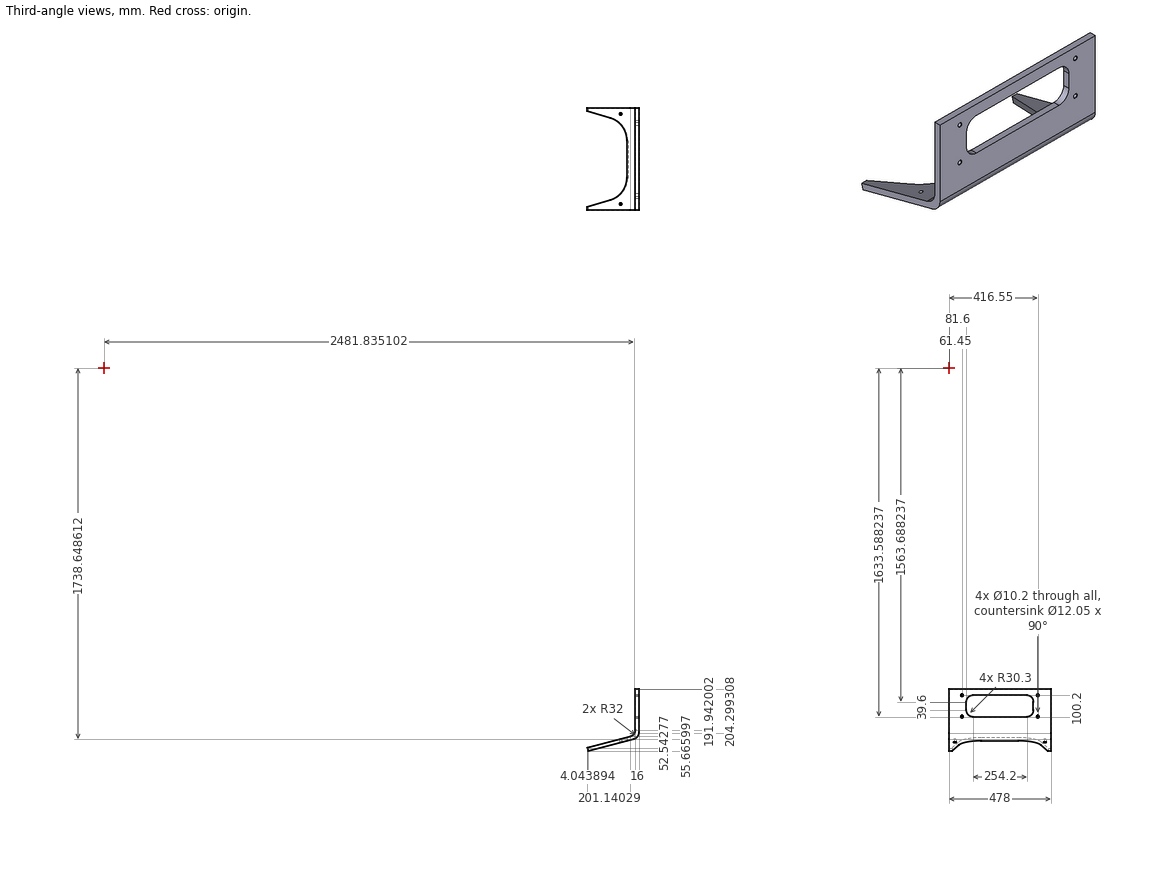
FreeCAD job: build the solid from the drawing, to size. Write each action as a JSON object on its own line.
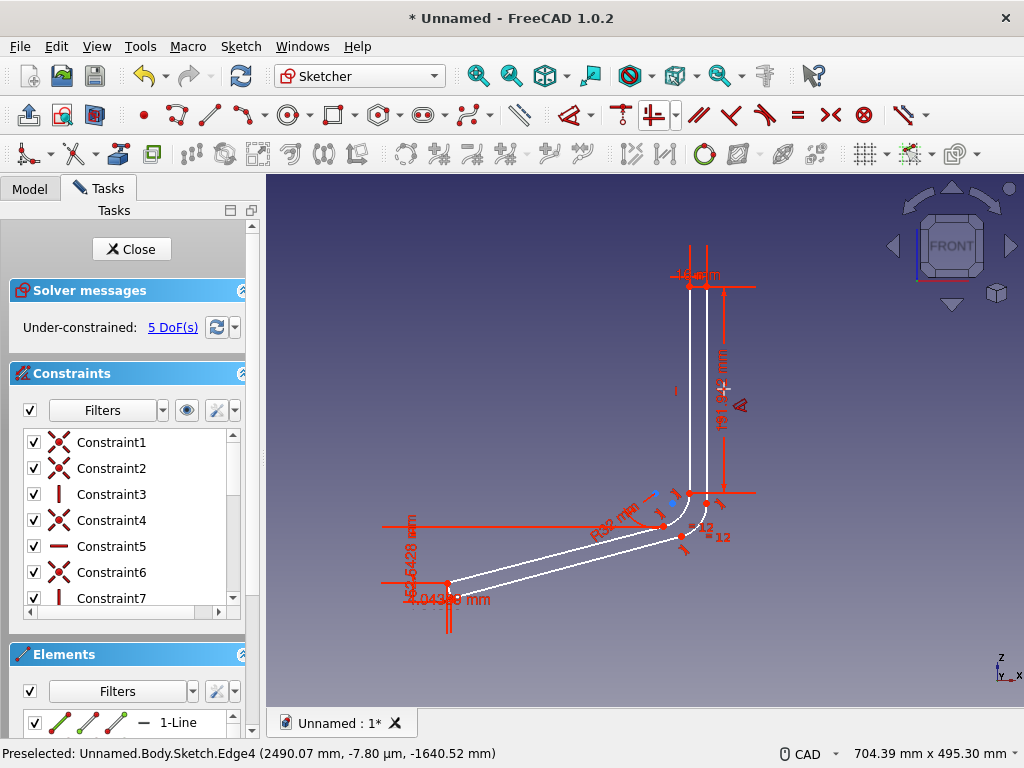
{"action": "left_click", "coordinate": [707, 352]}
{"action": "left_click", "coordinate": [741, 345]}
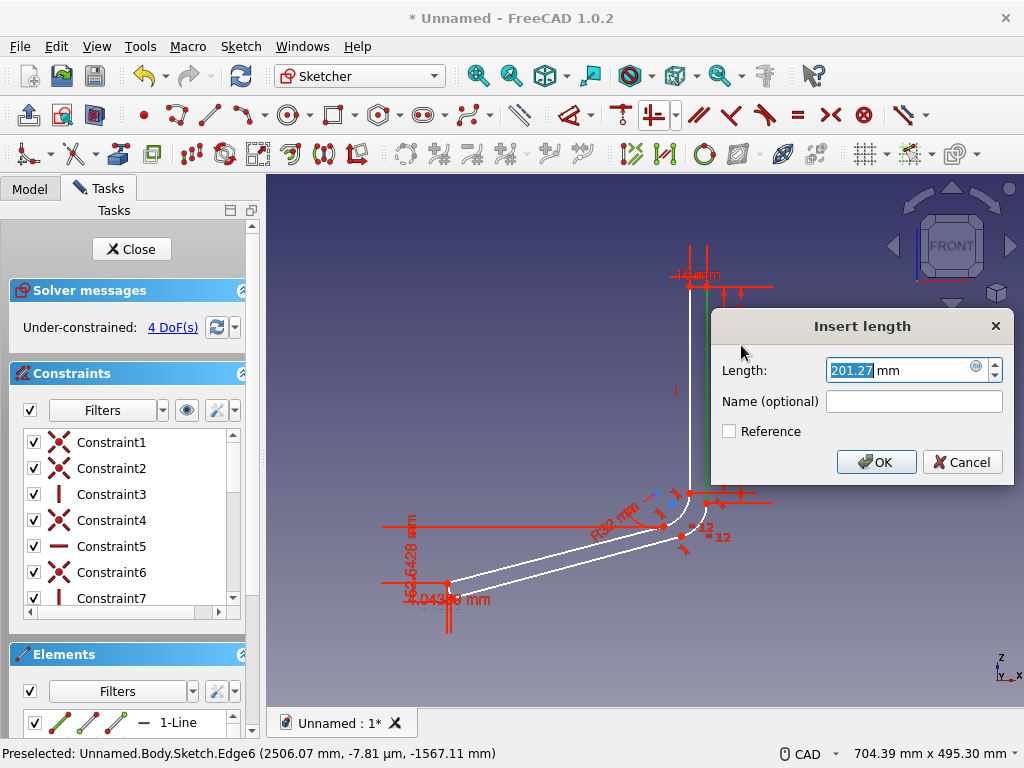
{"action": "type", "text": "204.299308"}
{"action": "key", "text": "Return"}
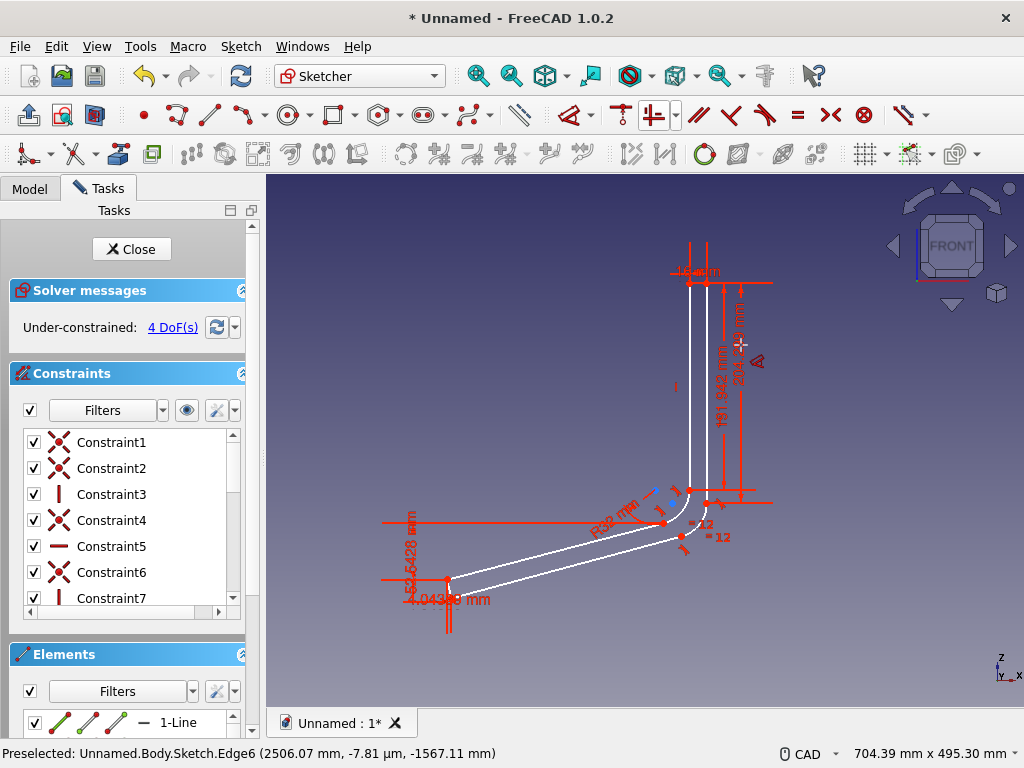
{"action": "left_click", "coordinate": [612, 555]}
{"action": "left_click", "coordinate": [715, 567]}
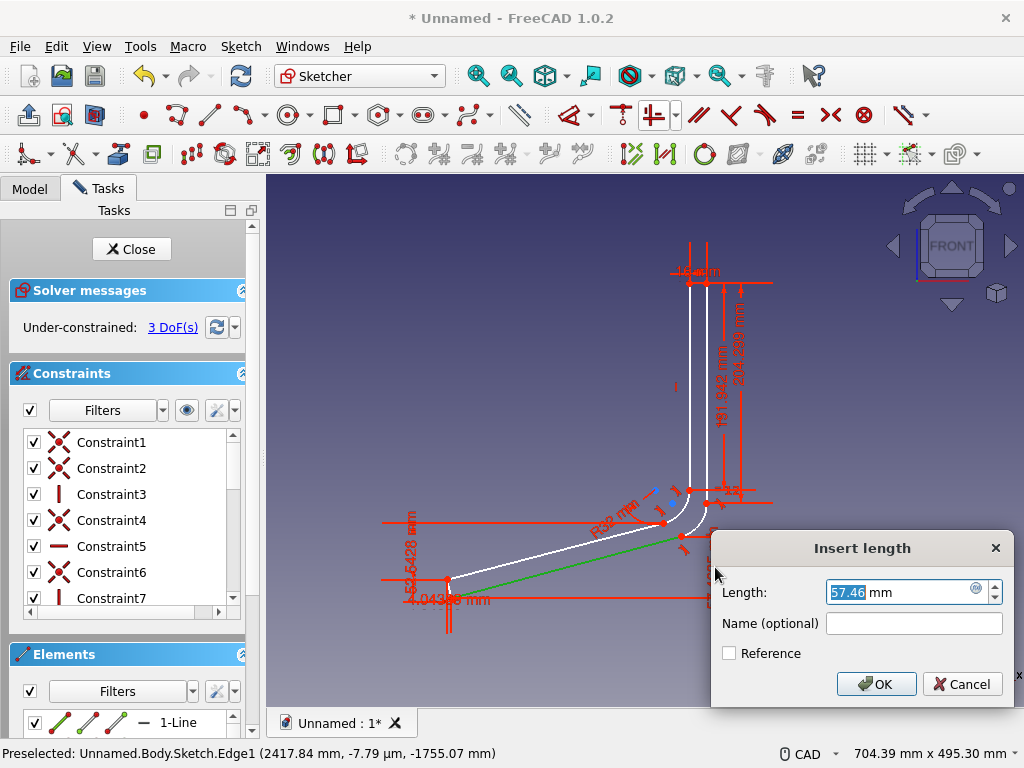
{"action": "type", "text": "55.665997"}
{"action": "key", "text": "Return"}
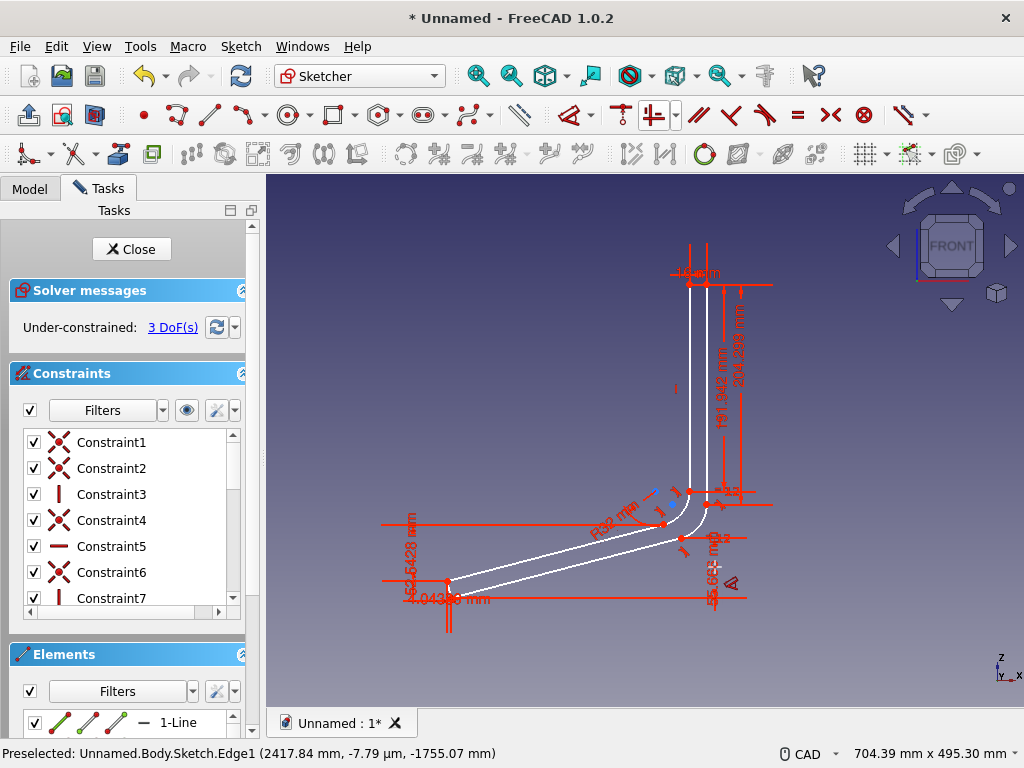
{"action": "left_click", "coordinate": [512, 564]}
{"action": "left_click", "coordinate": [555, 615]}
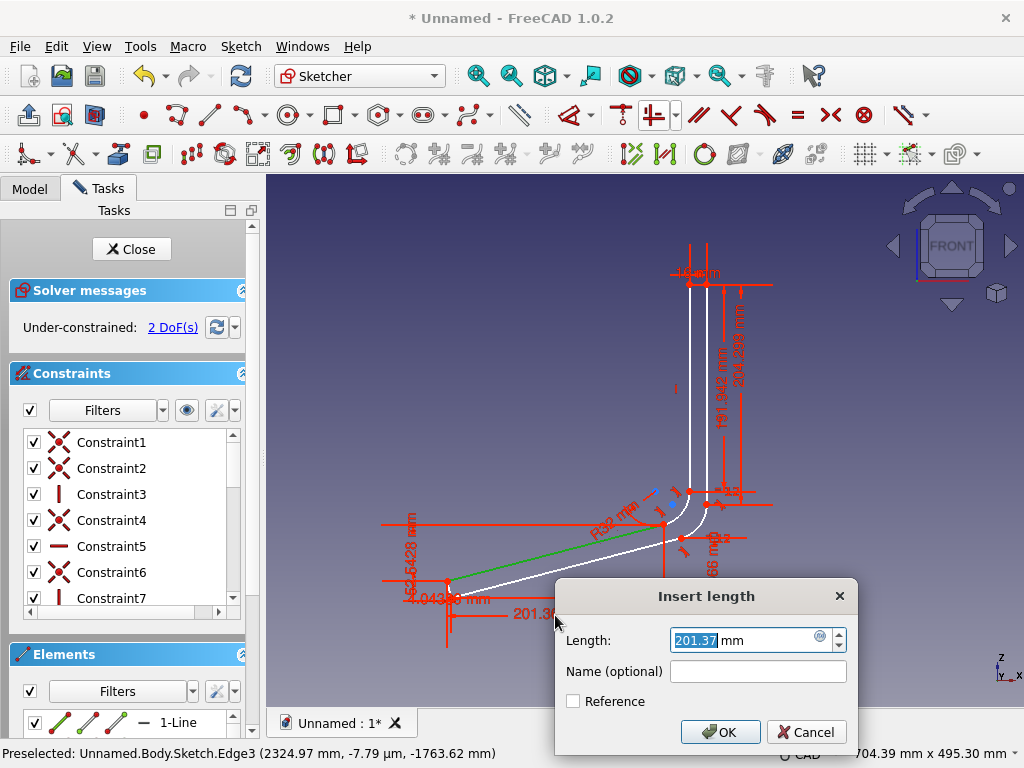
{"action": "type", "text": "201.14029"}
{"action": "key", "text": "Return"}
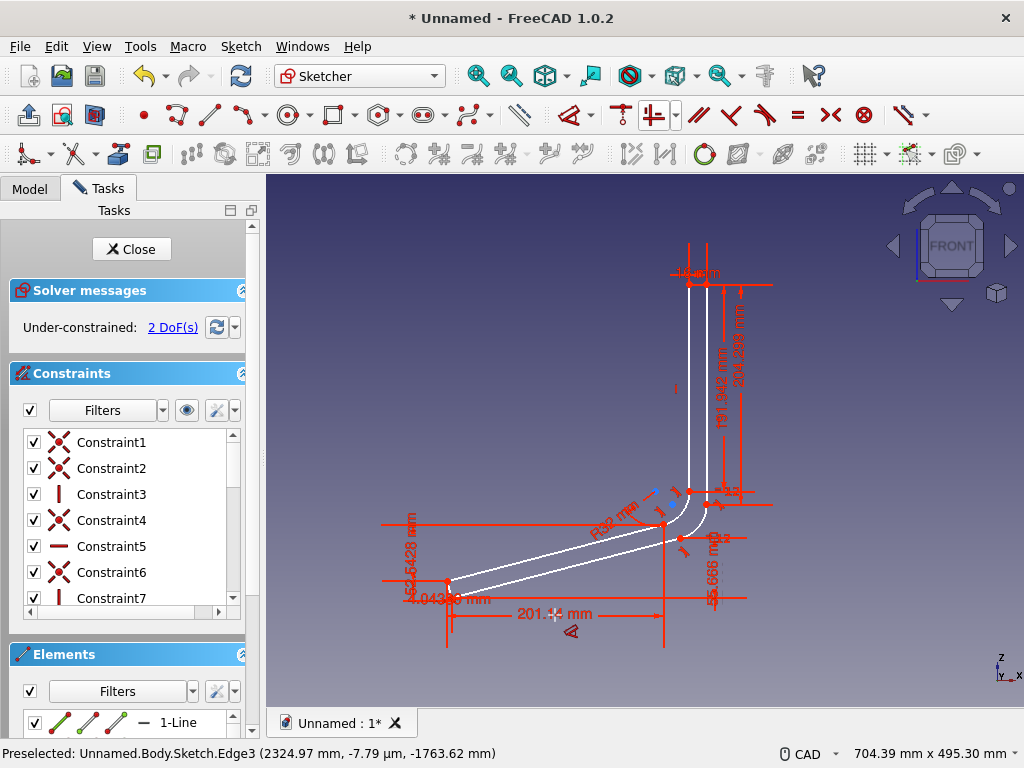
{"action": "left_click", "coordinate": [681, 538]}
{"action": "left_click", "coordinate": [623, 572]}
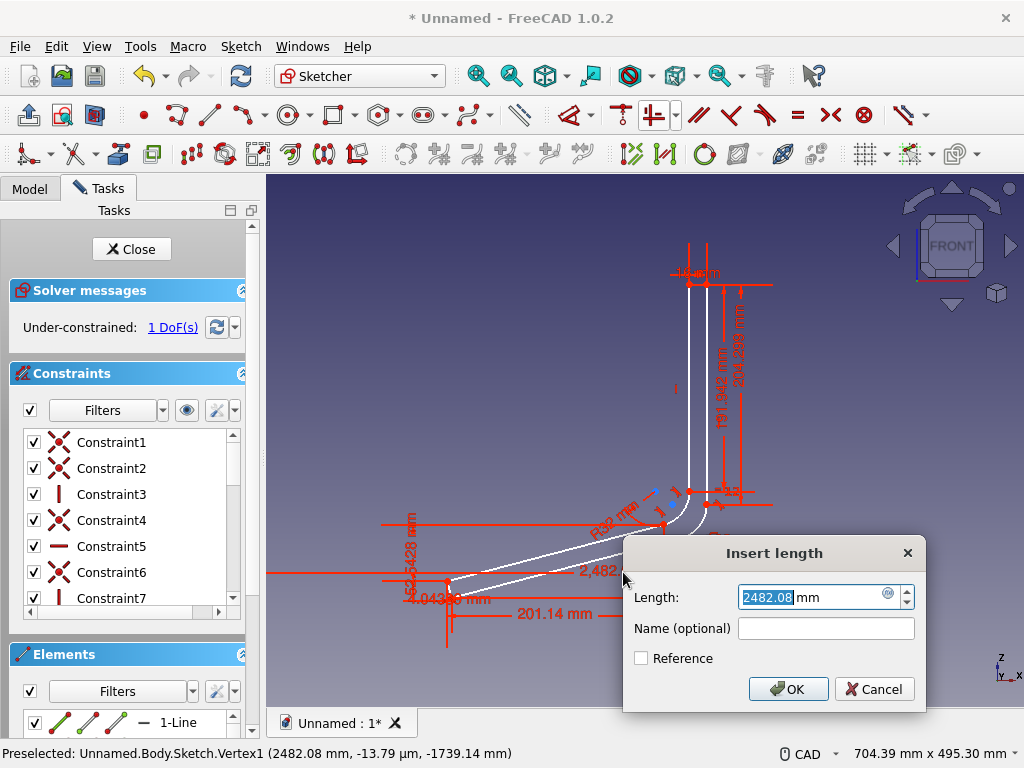
{"action": "type", "text": "2481.835102"}
{"action": "key", "text": "Return"}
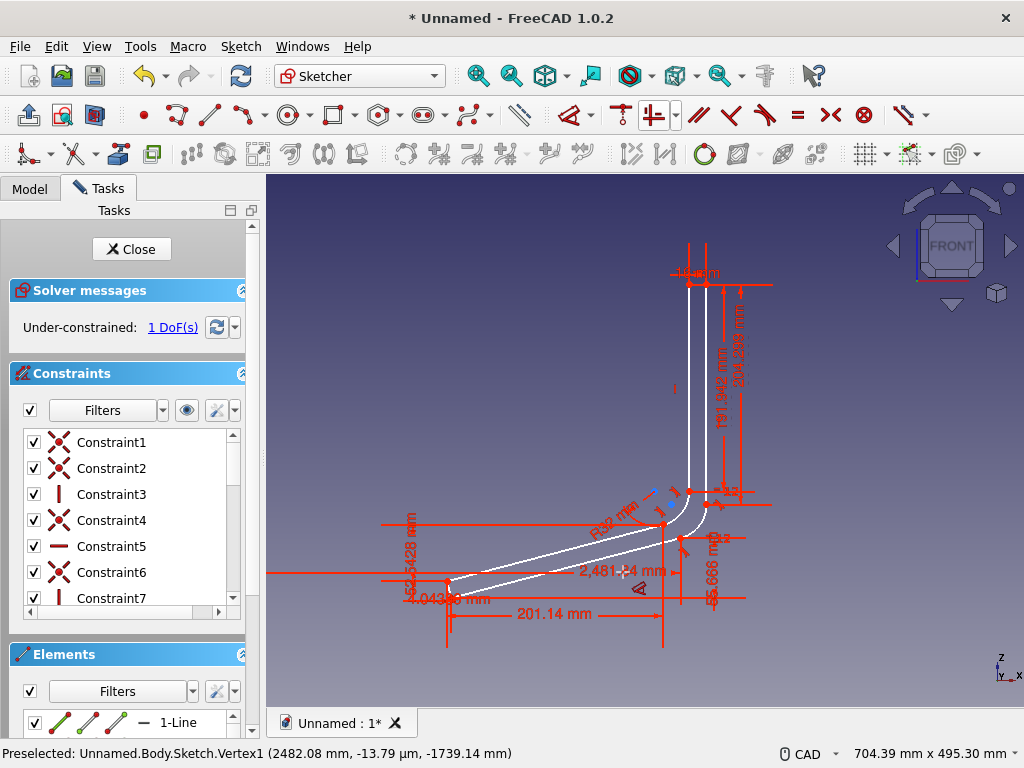
{"action": "left_click", "coordinate": [681, 538]}
{"action": "left_click", "coordinate": [715, 252]}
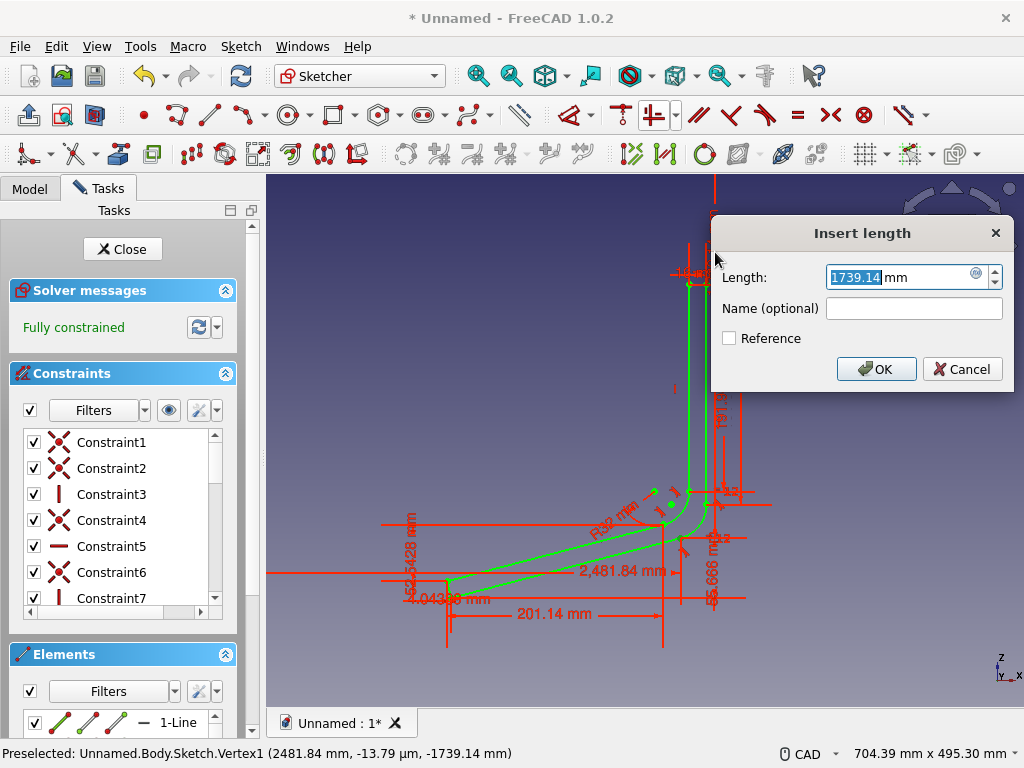
{"action": "type", "text": "1738.648612"}
{"action": "key", "text": "Return"}
{"action": "key", "text": "Escape"}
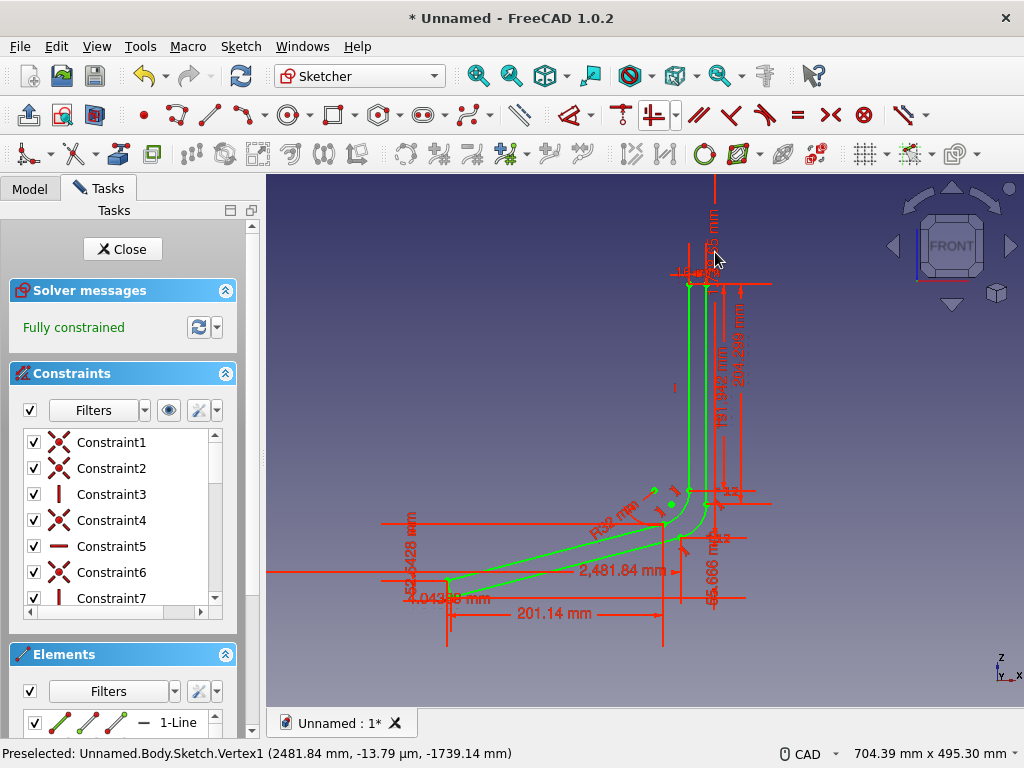
{"action": "left_click", "coordinate": [123, 249]}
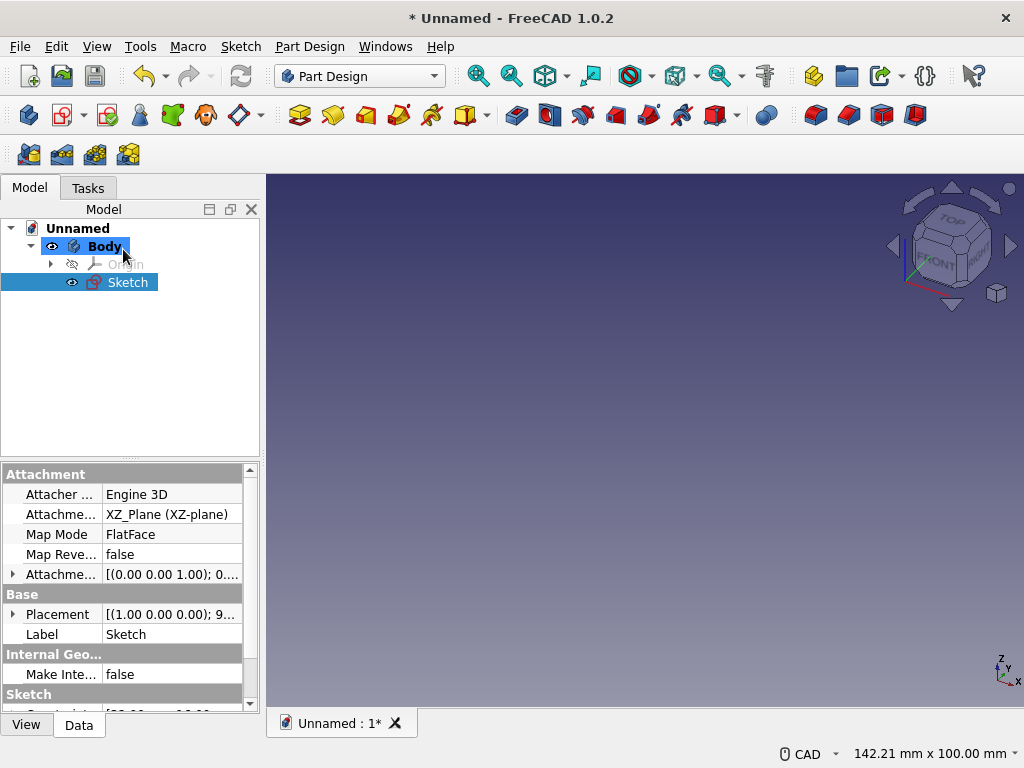
{"action": "left_click", "coordinate": [300, 116]}